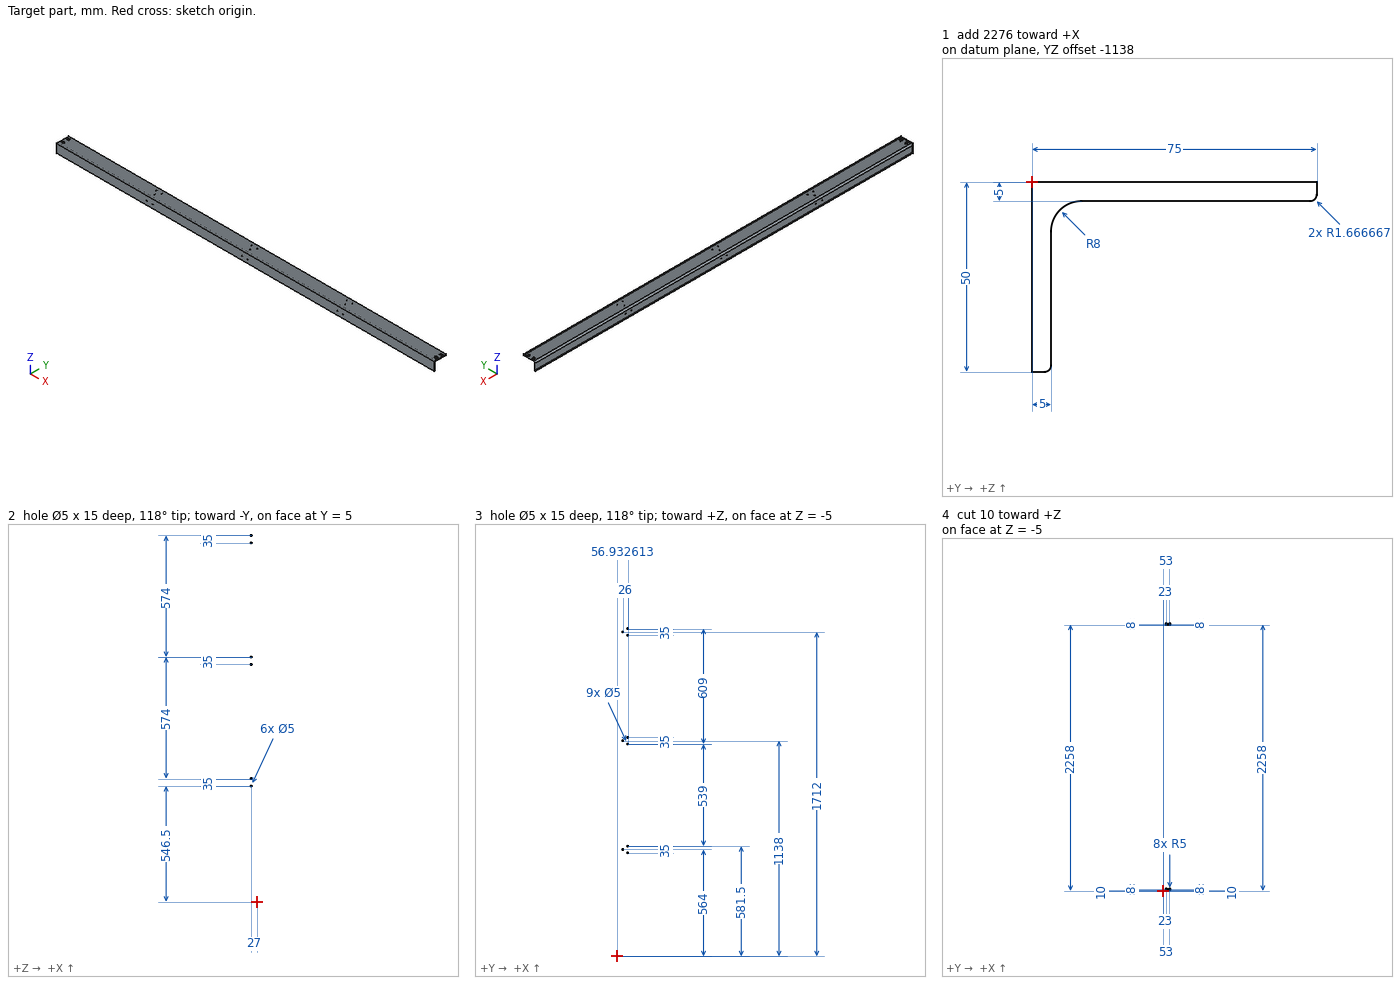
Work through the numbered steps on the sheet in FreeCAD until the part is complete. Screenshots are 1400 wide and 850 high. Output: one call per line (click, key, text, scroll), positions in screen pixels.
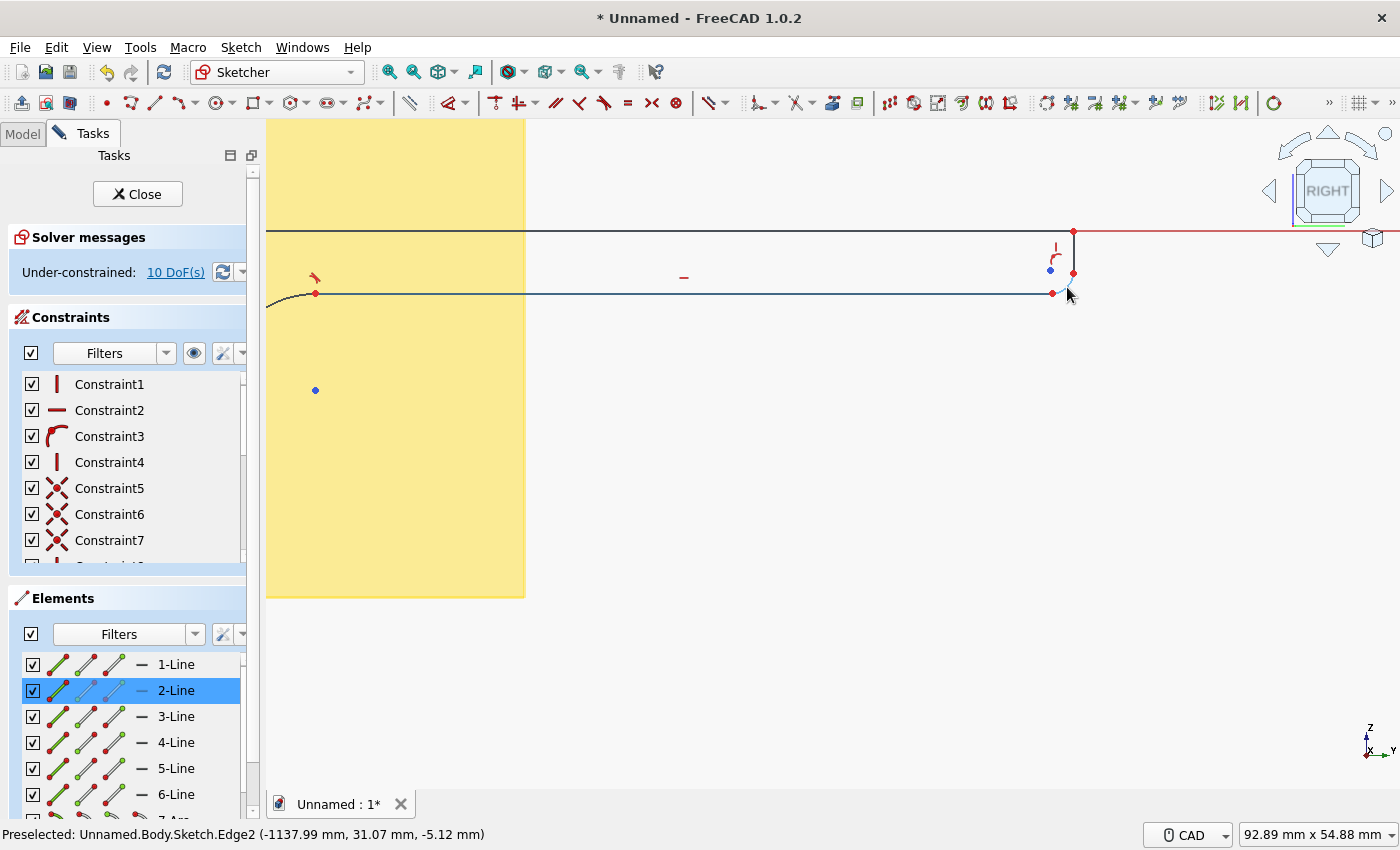
click(1067, 287)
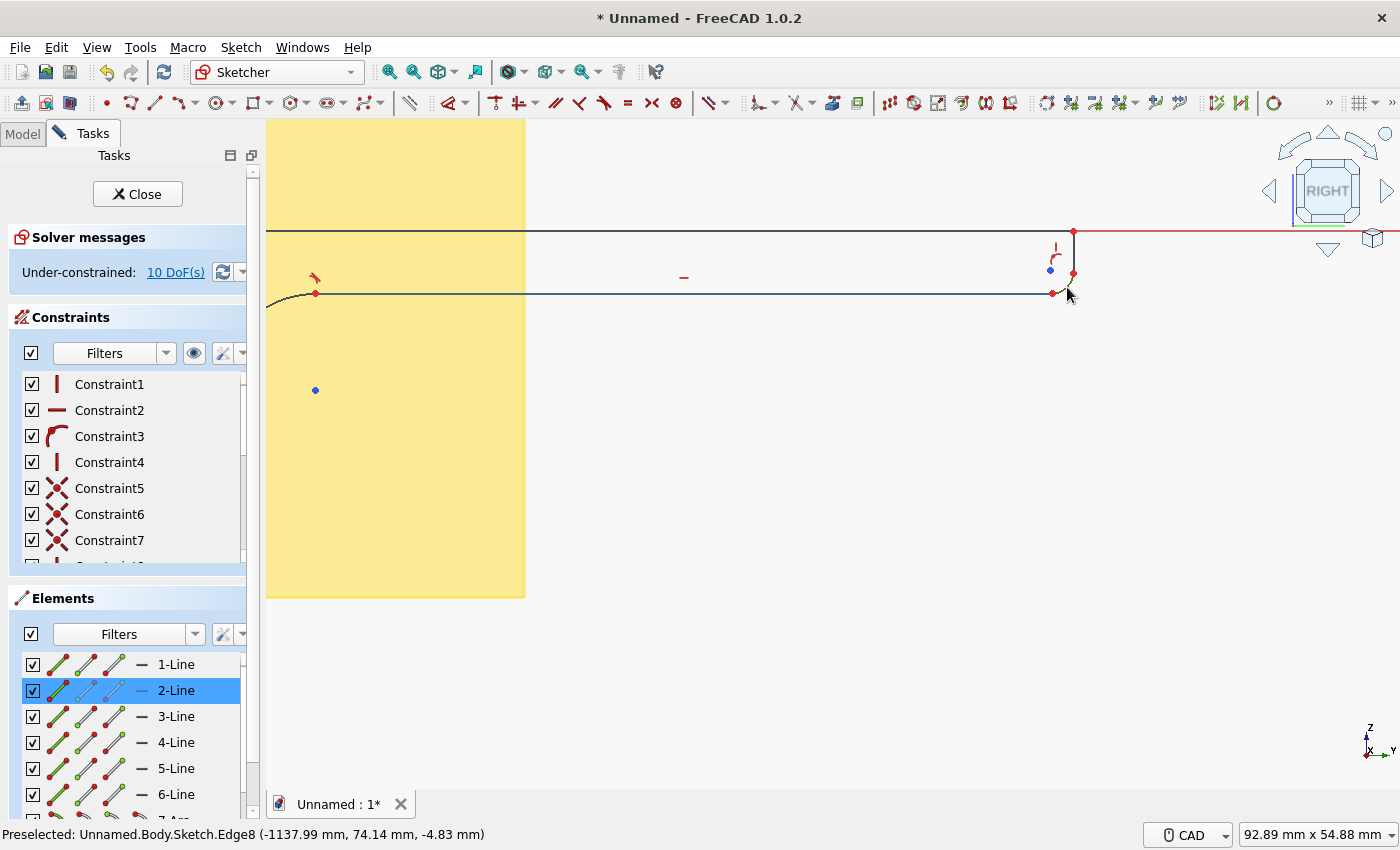
click(604, 104)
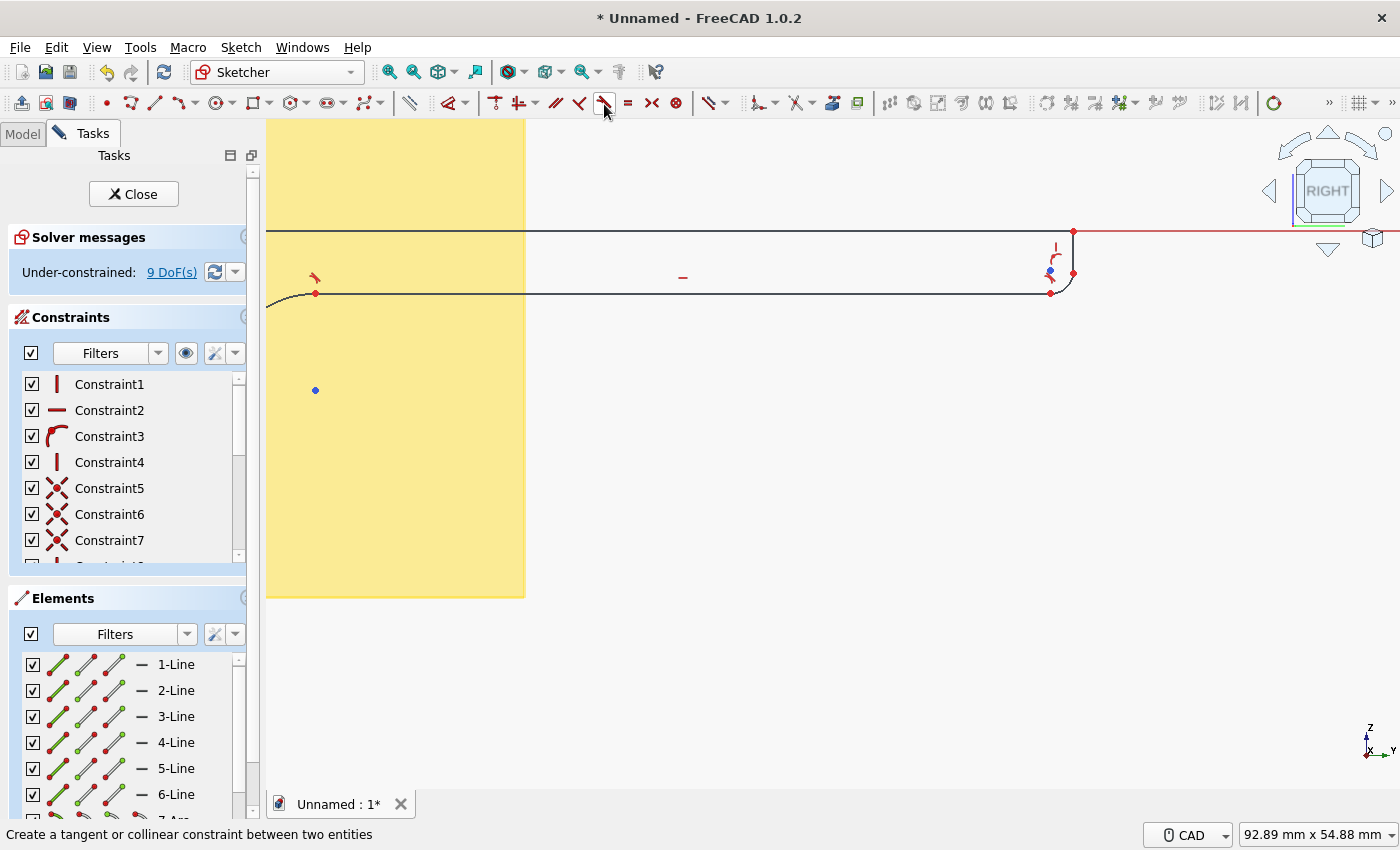
click(1073, 261)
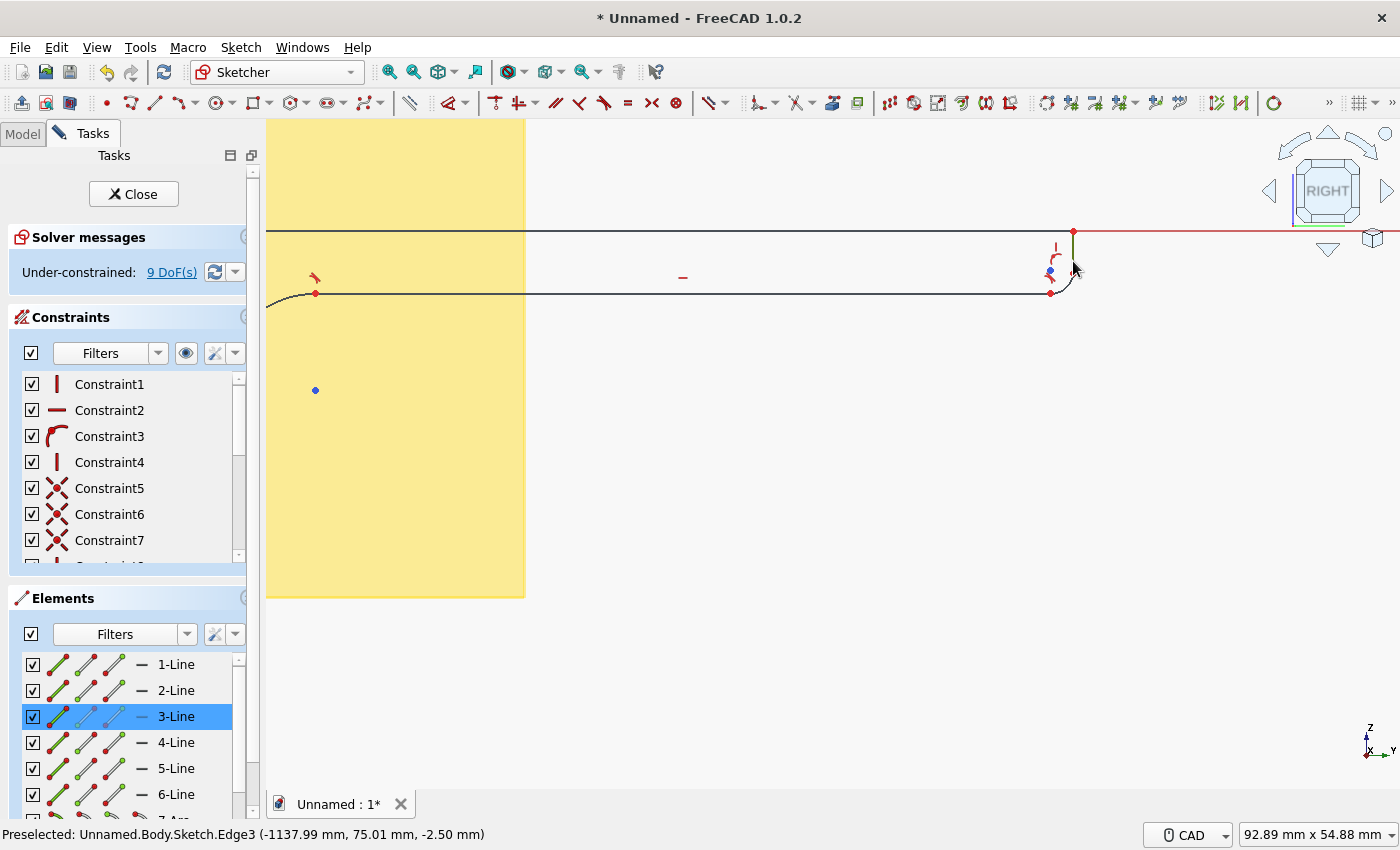
scroll(1060, 292, up, 2)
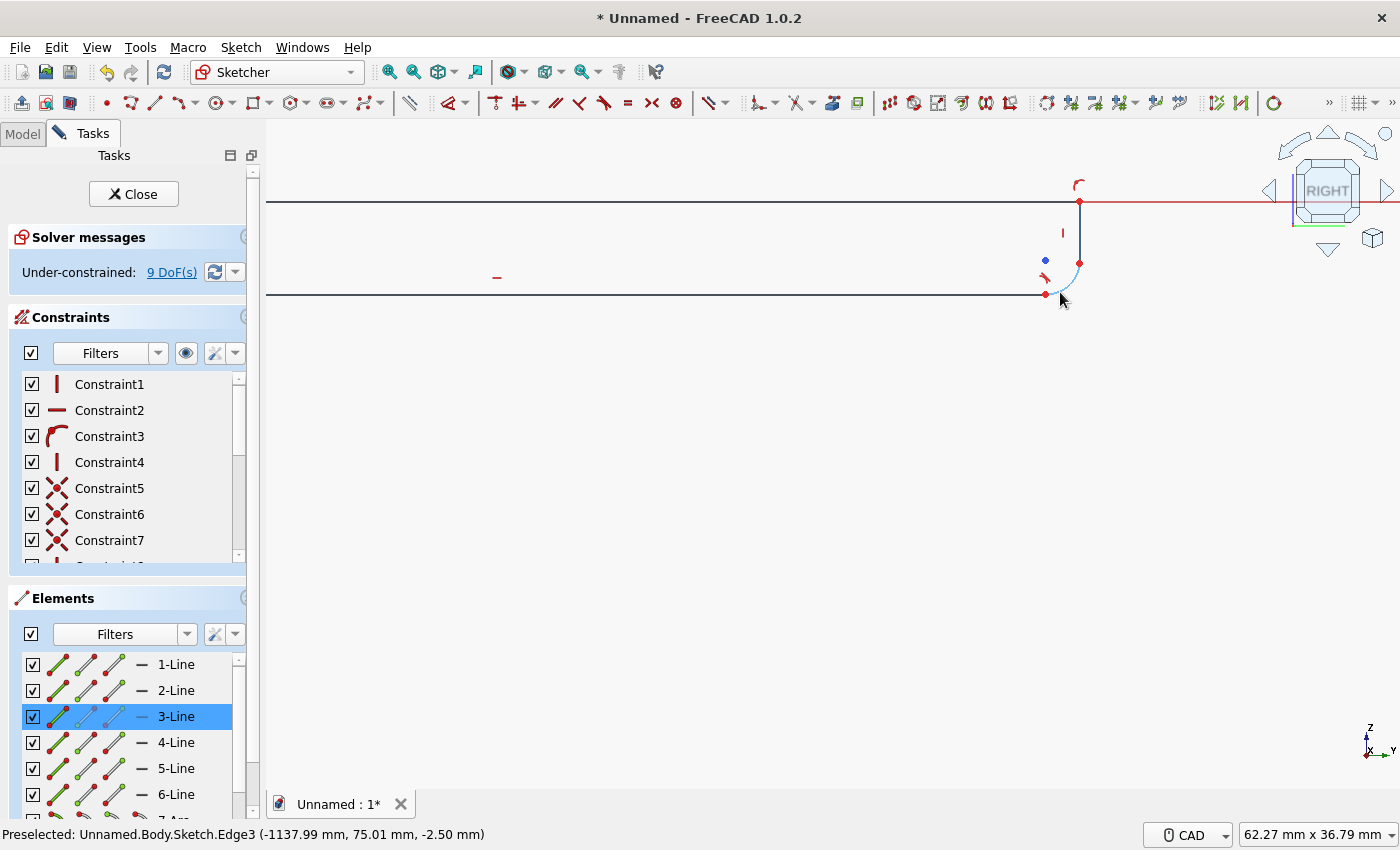
click(1060, 291)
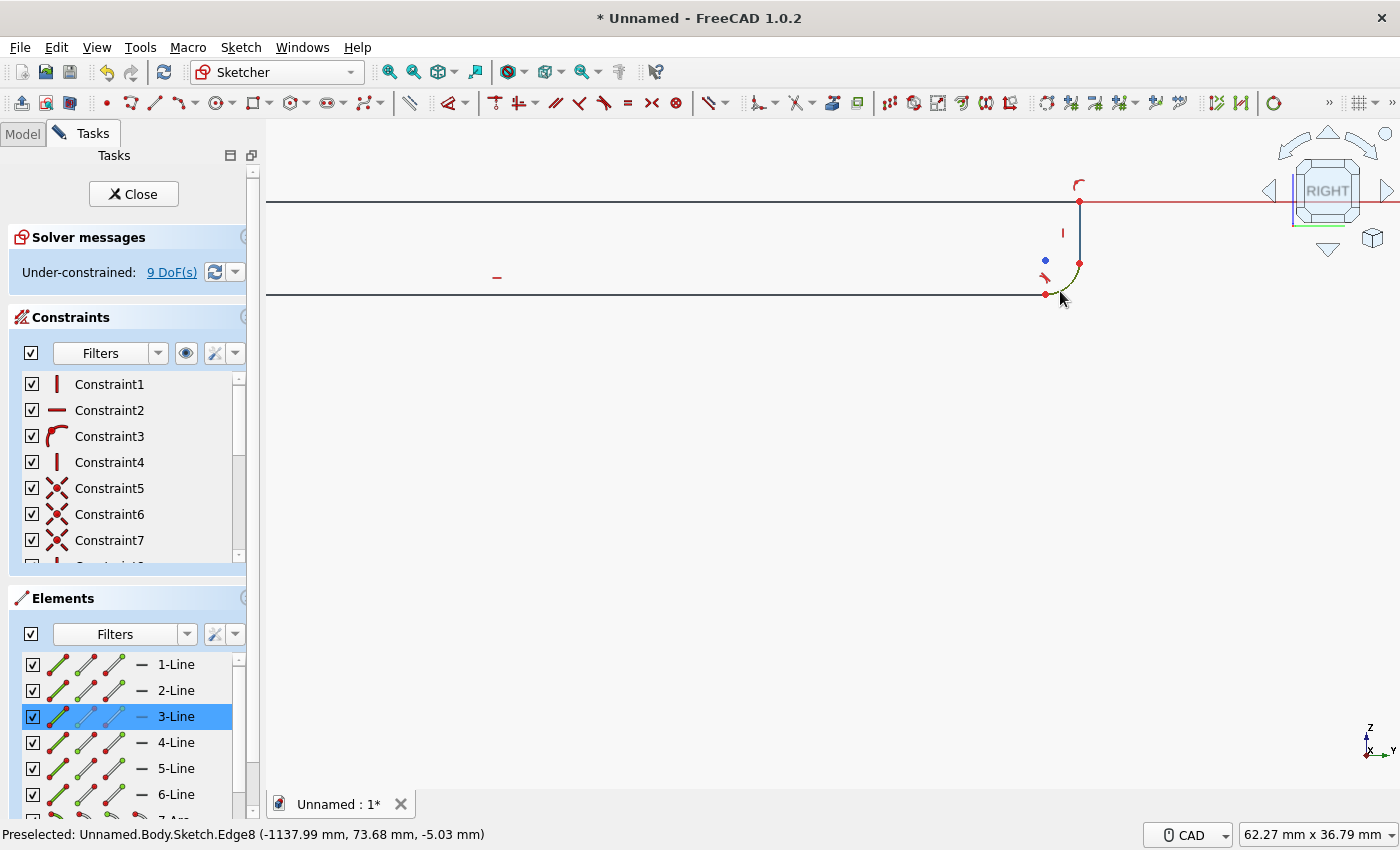
click(604, 104)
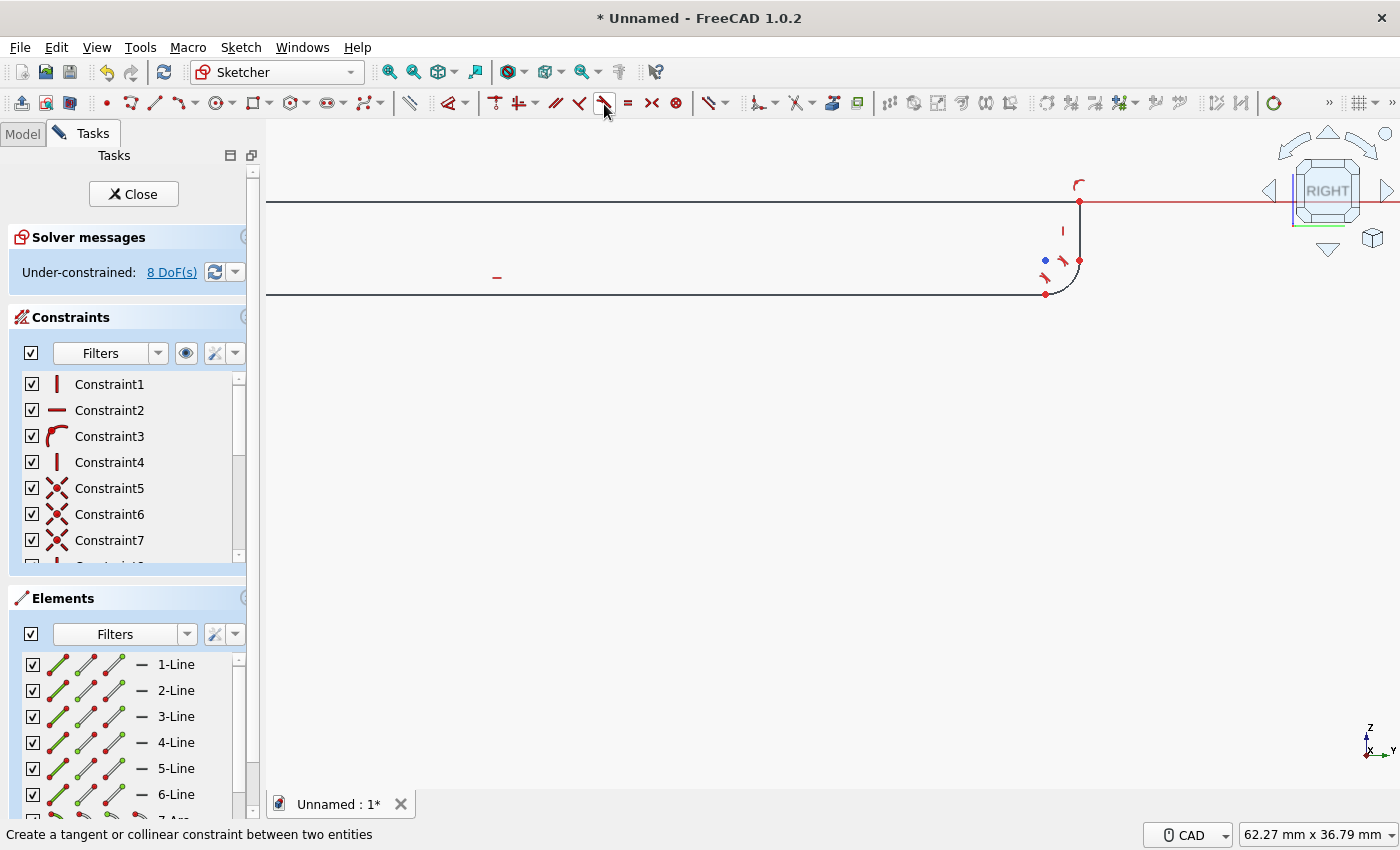
scroll(1065, 288, down, 4)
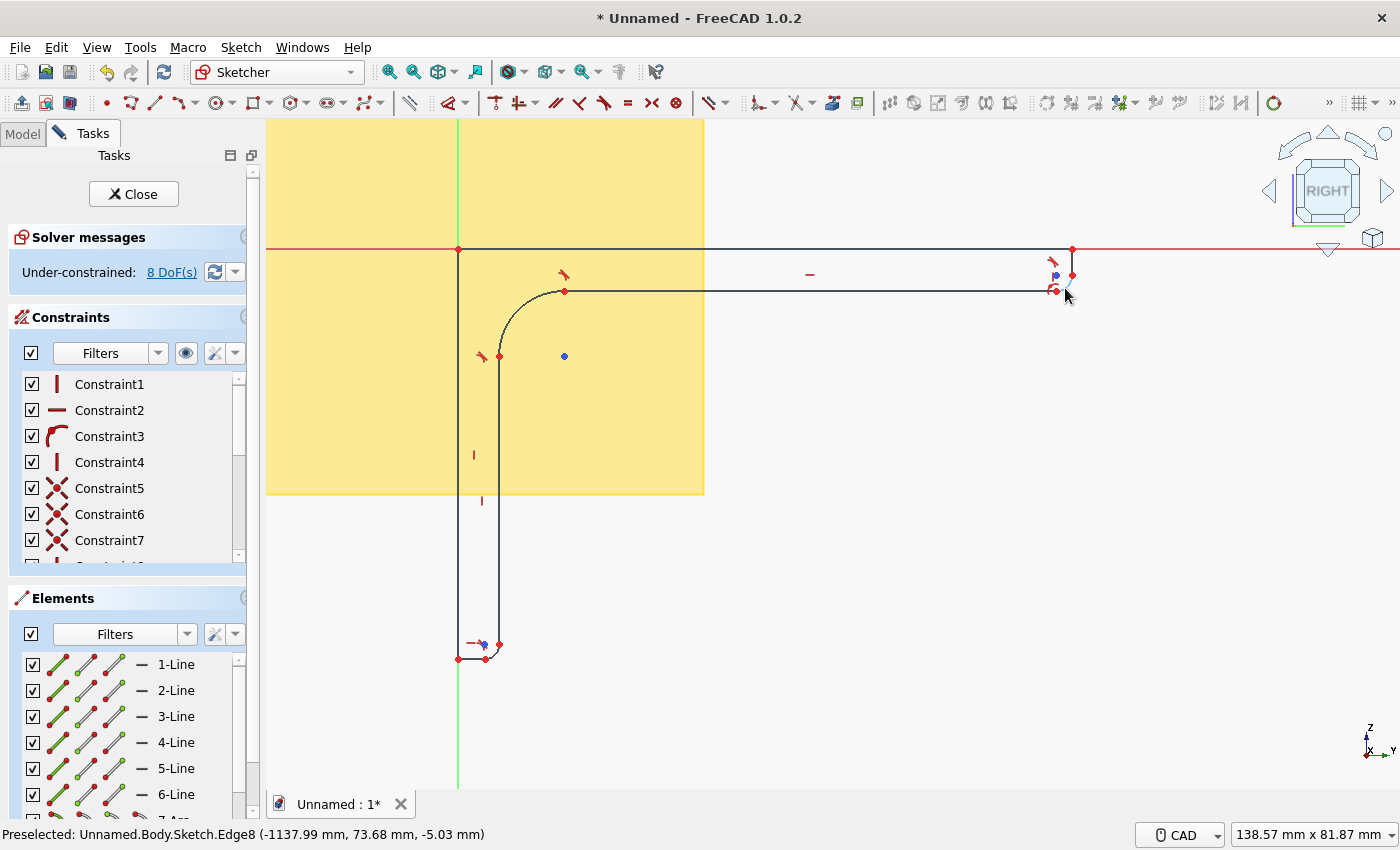
scroll(466, 659, up, 3)